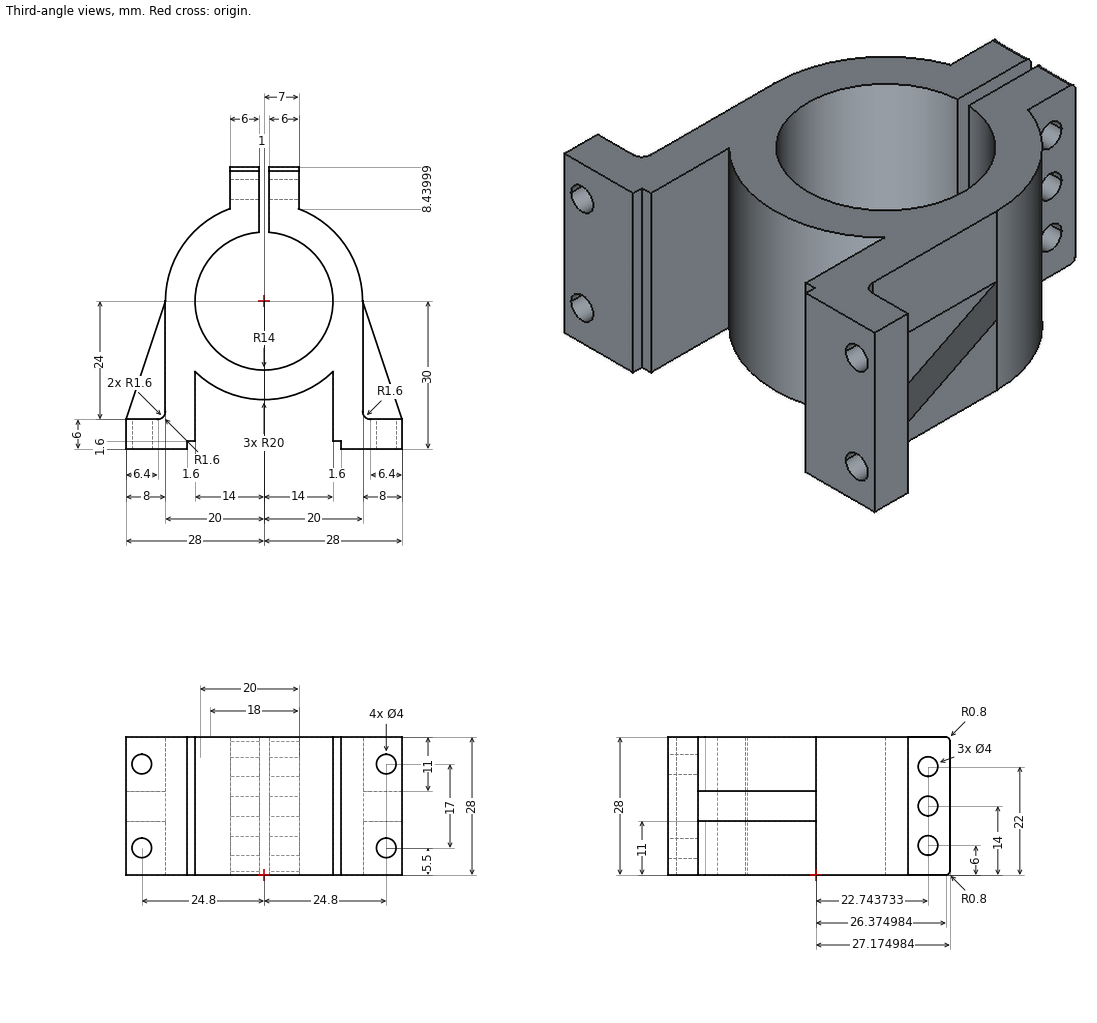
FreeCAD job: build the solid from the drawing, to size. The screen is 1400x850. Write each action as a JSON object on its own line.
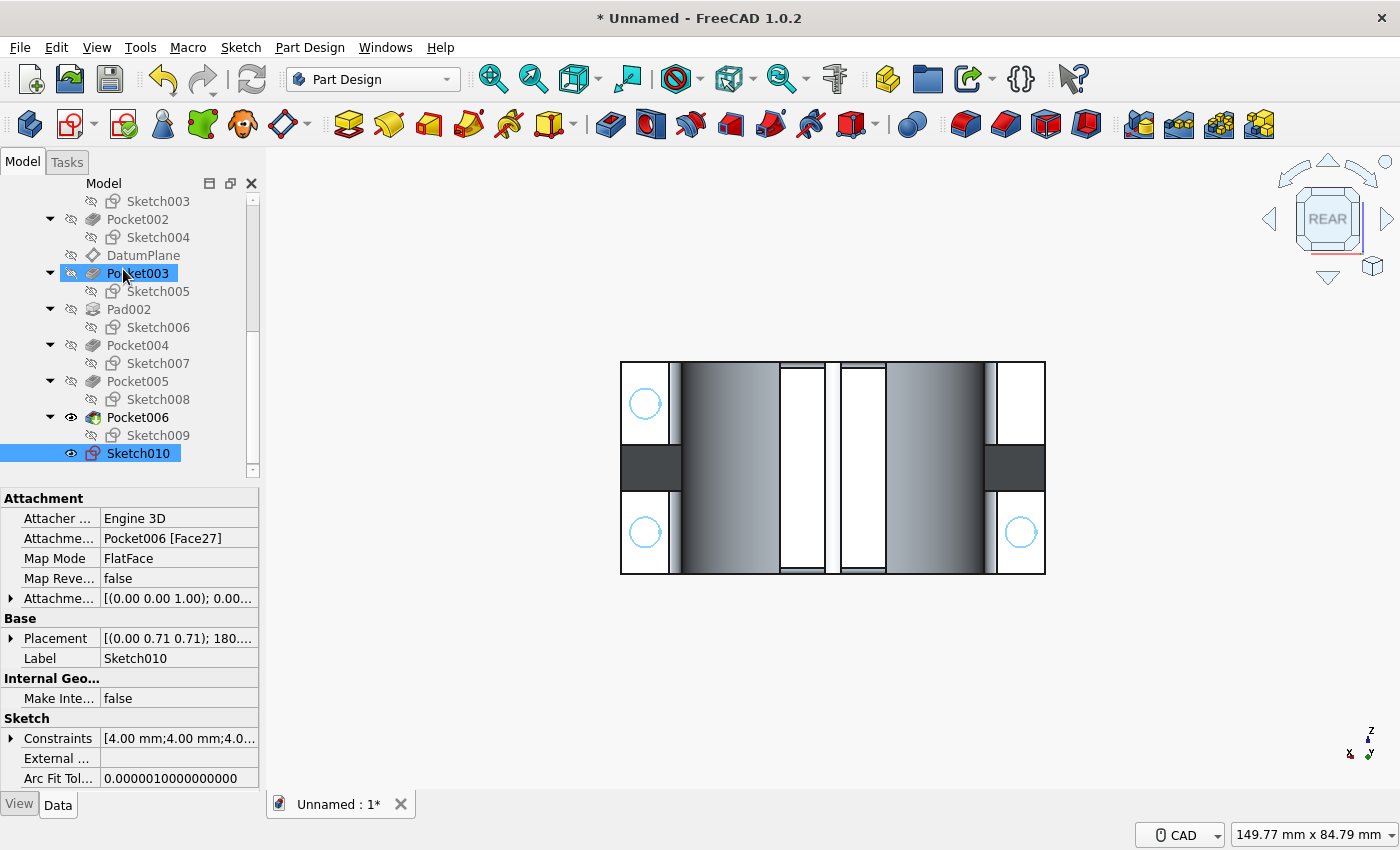
{"action": "left_click", "coordinate": [612, 124]}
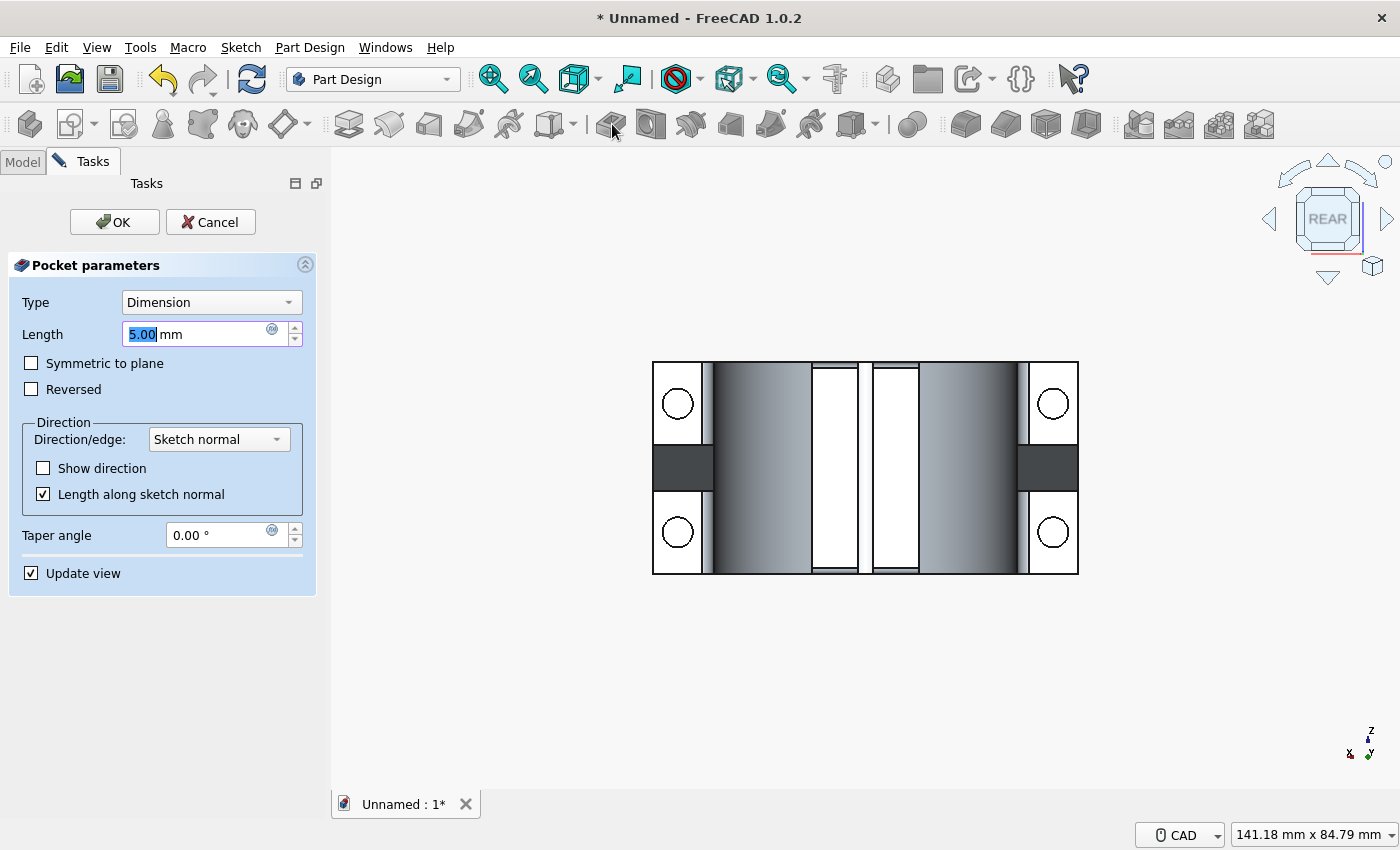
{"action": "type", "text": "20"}
{"action": "key", "text": "Tab"}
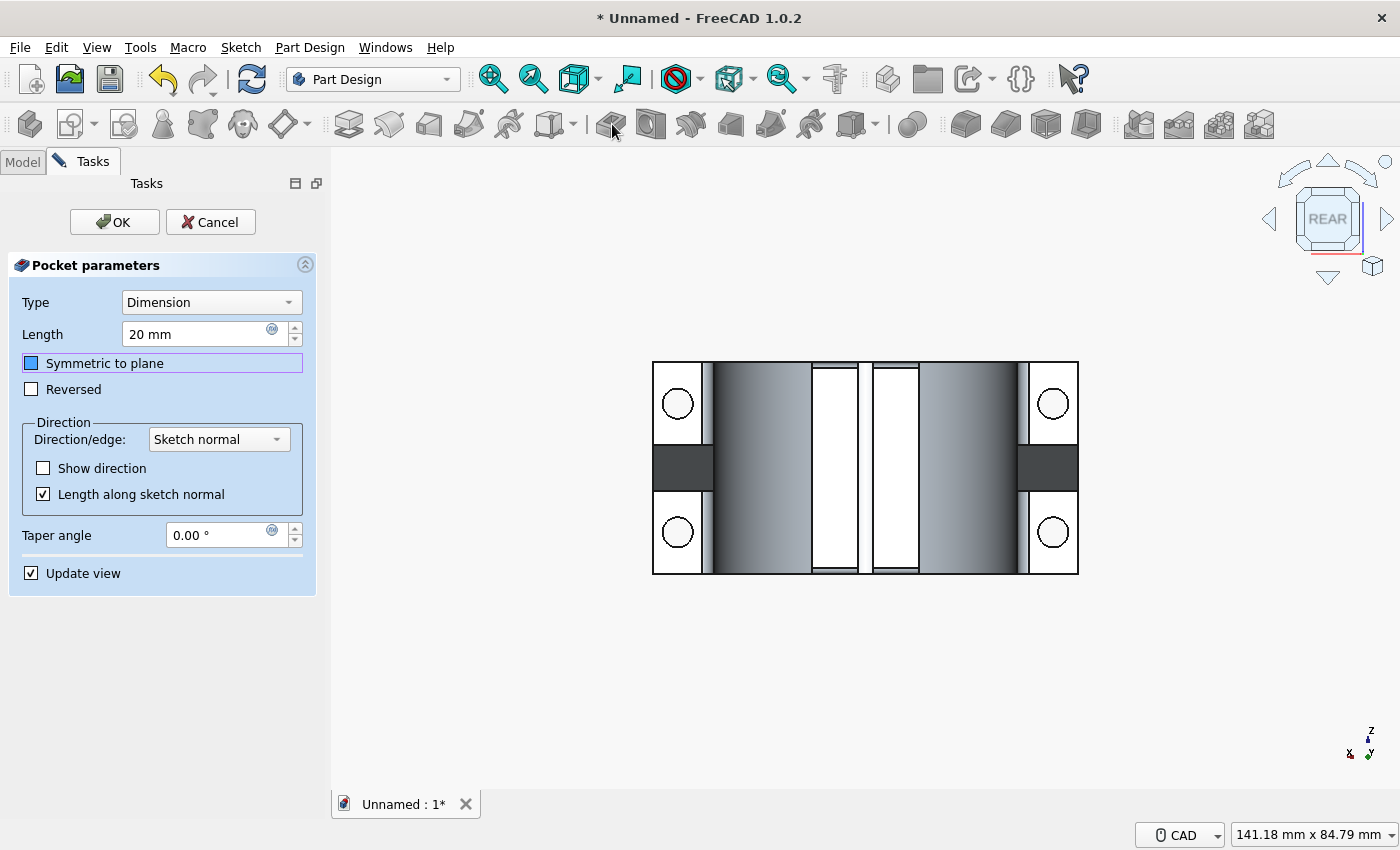
{"action": "left_click", "coordinate": [115, 222]}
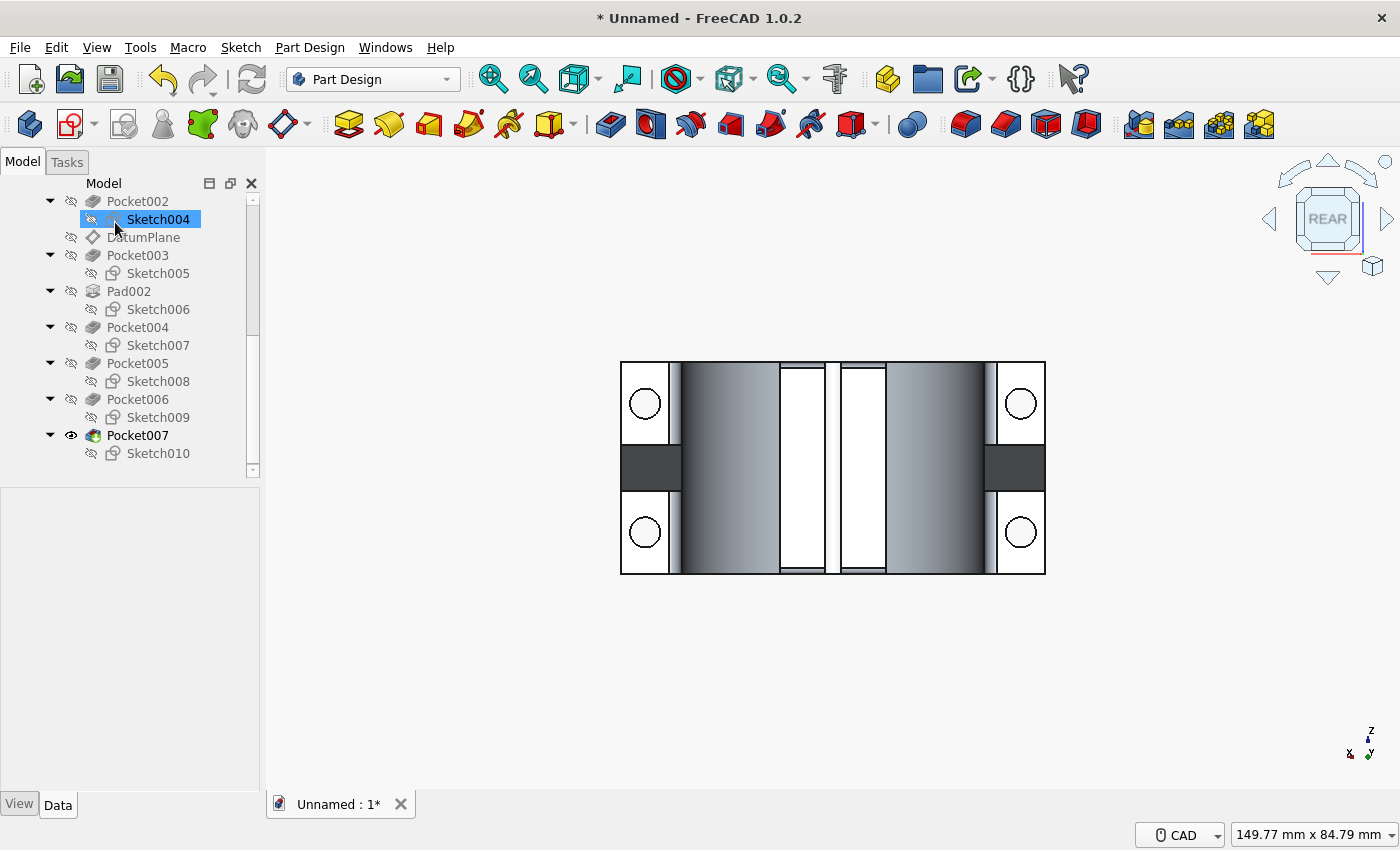
{"action": "key", "text": "0"}